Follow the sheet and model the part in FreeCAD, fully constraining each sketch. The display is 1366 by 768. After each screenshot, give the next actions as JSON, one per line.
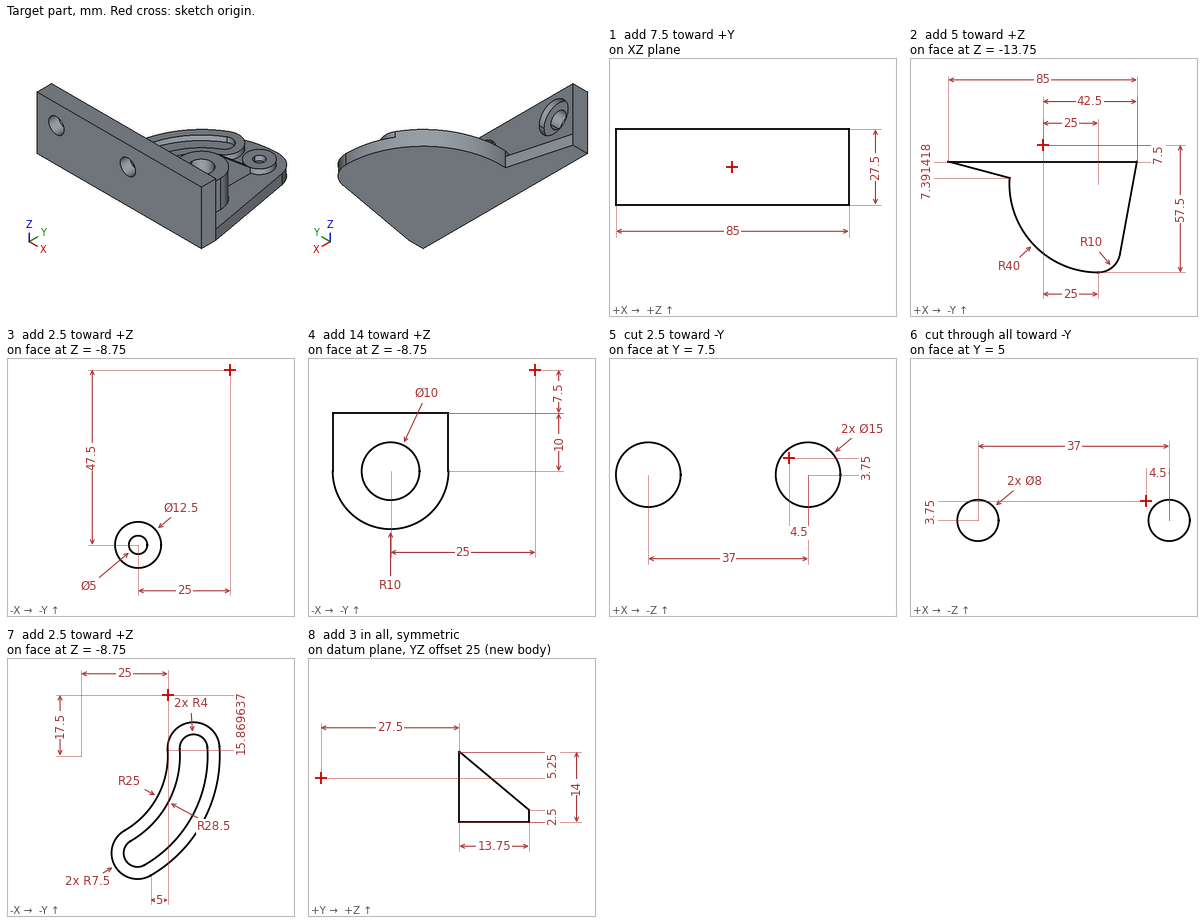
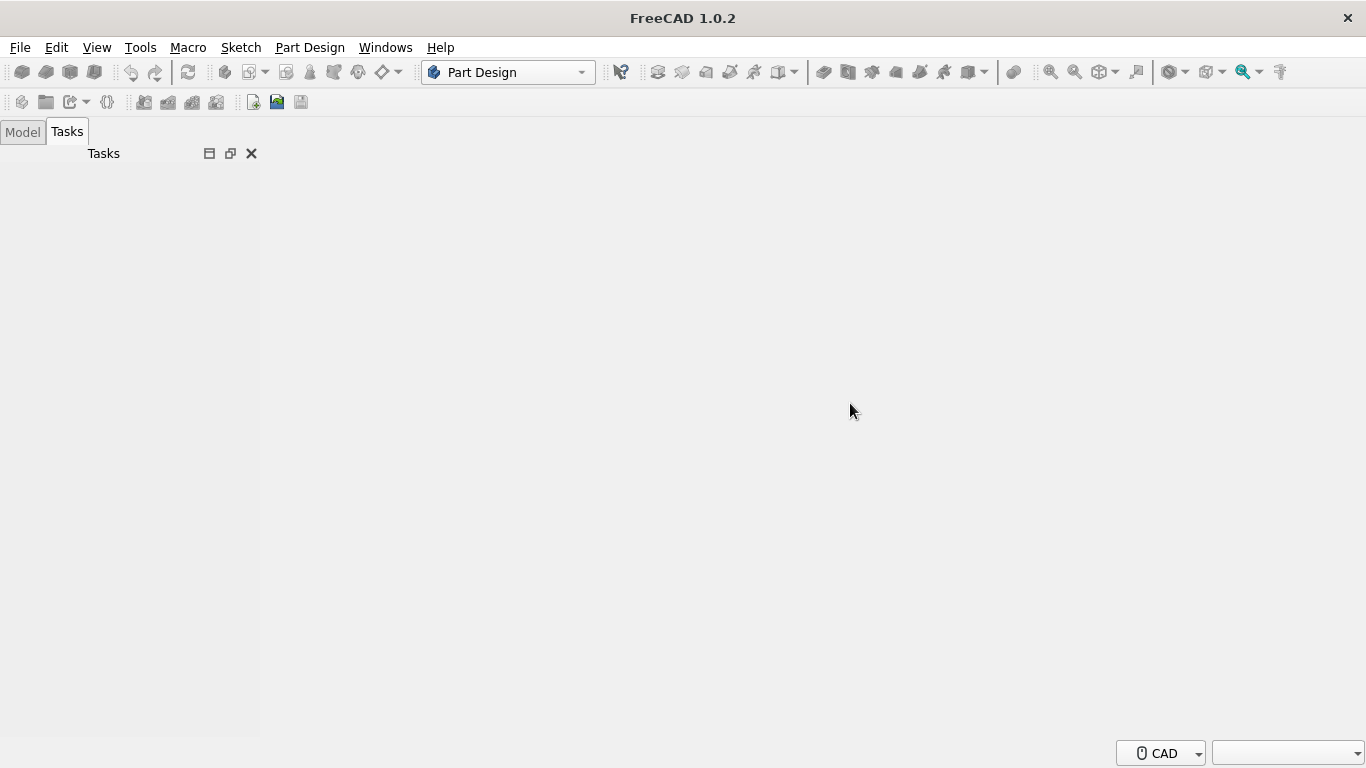
{"action": "left_click", "coordinate": [254, 102]}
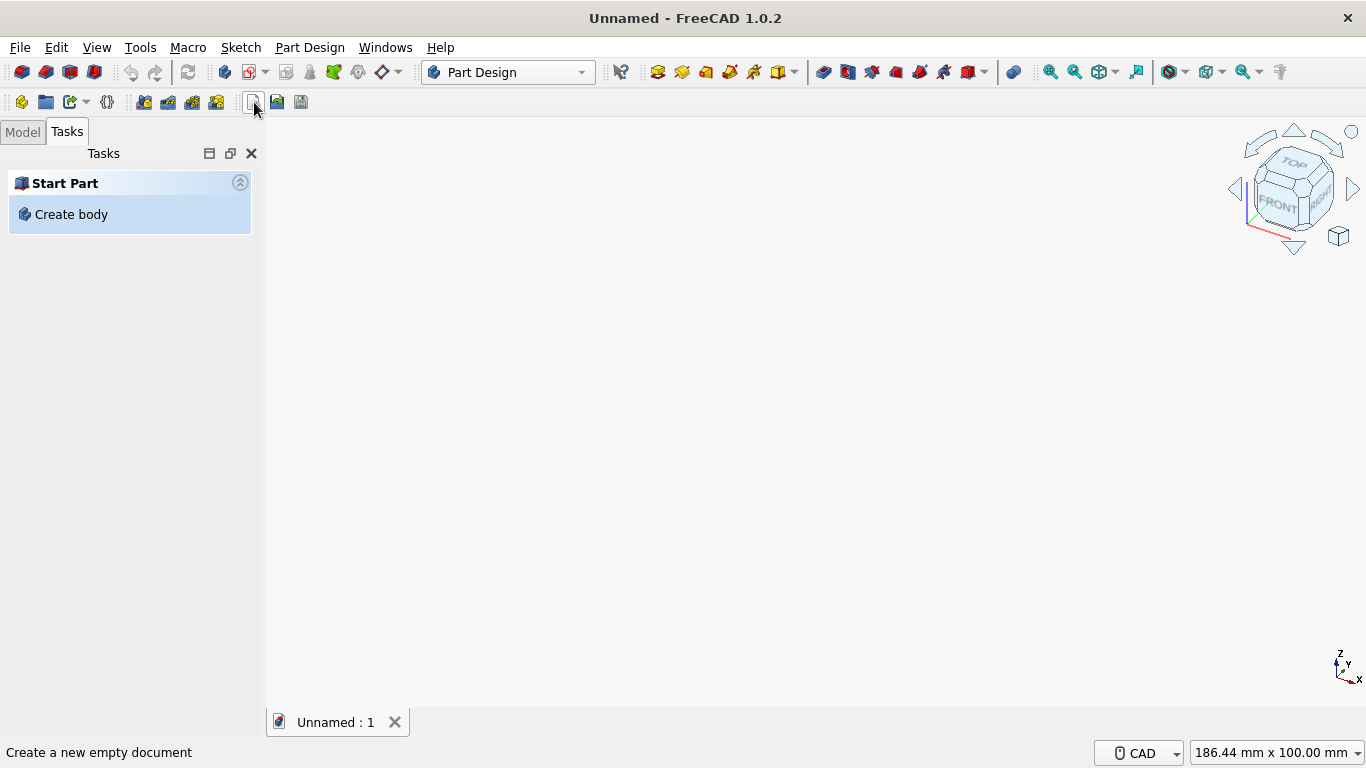
{"action": "left_click", "coordinate": [250, 72]}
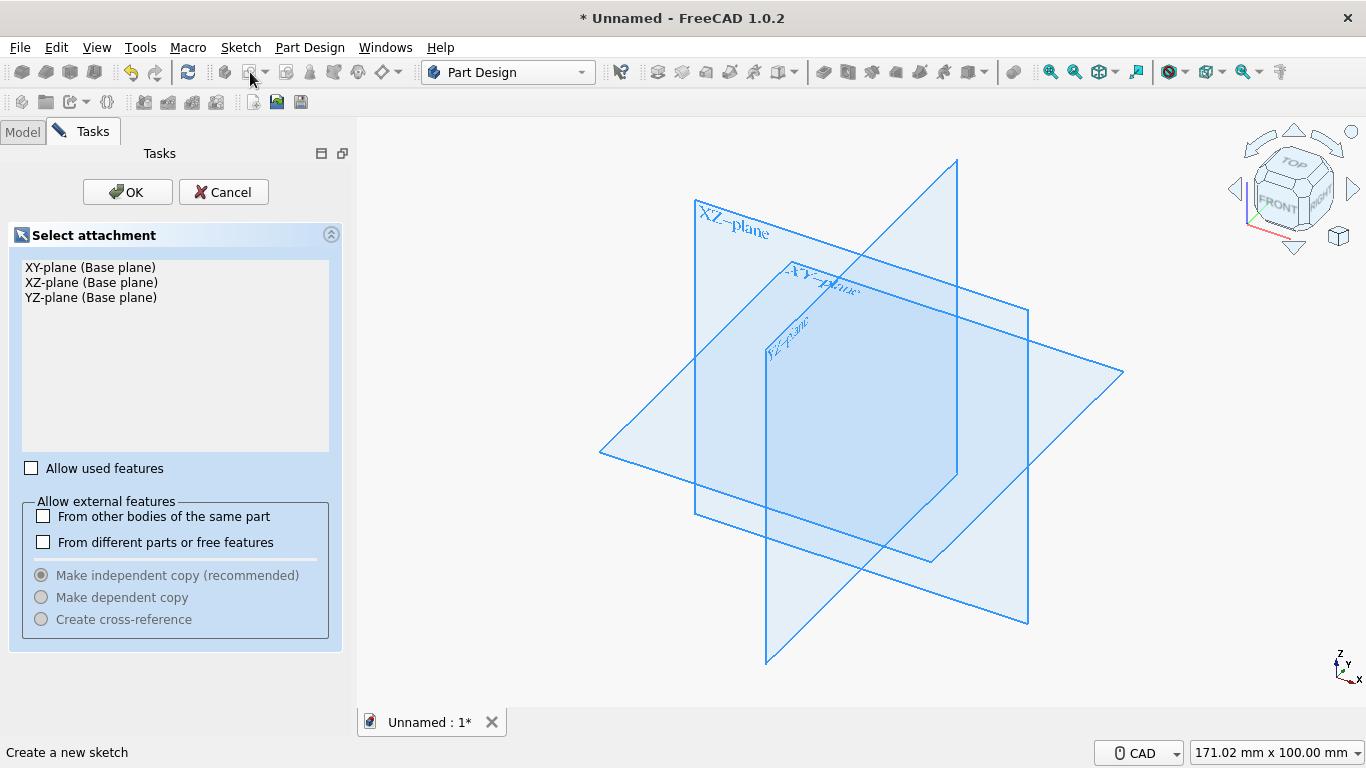
{"action": "left_click", "coordinate": [82, 282]}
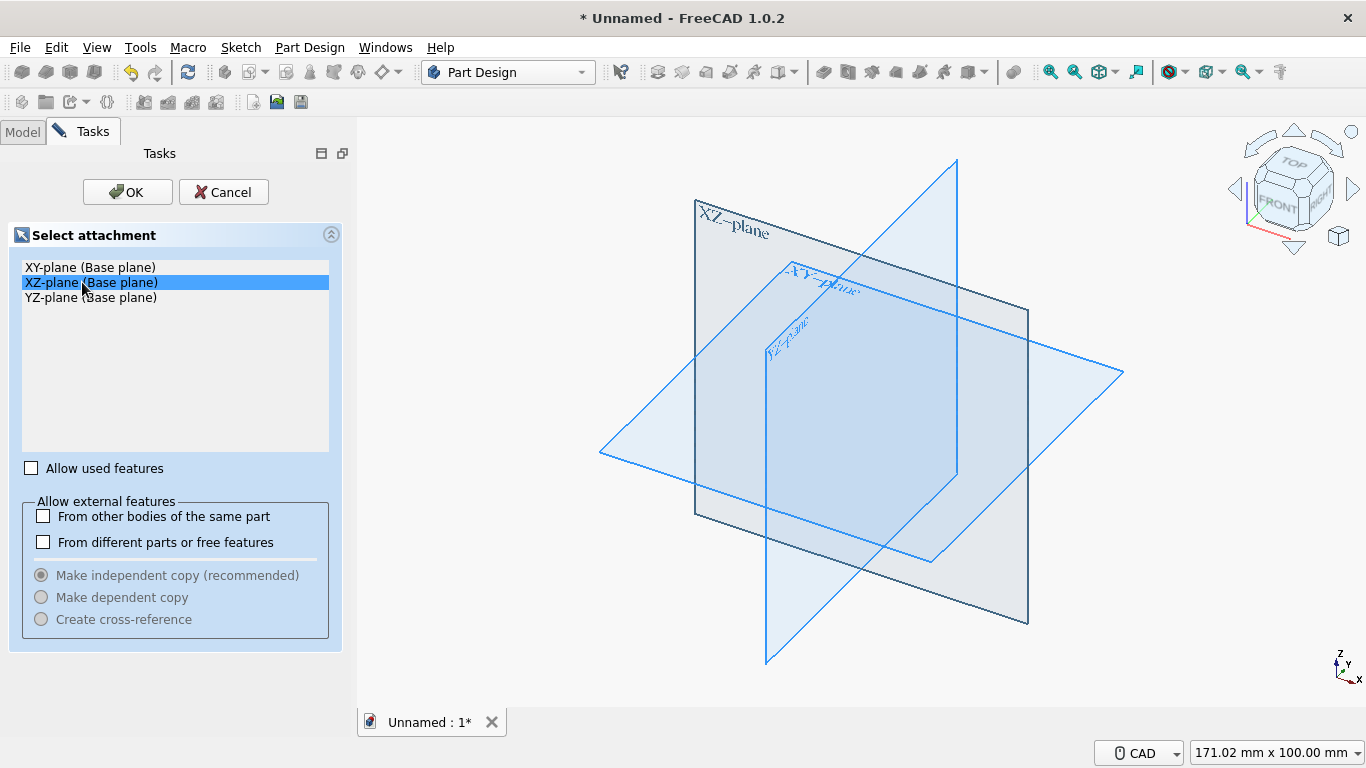
{"action": "left_click", "coordinate": [128, 192]}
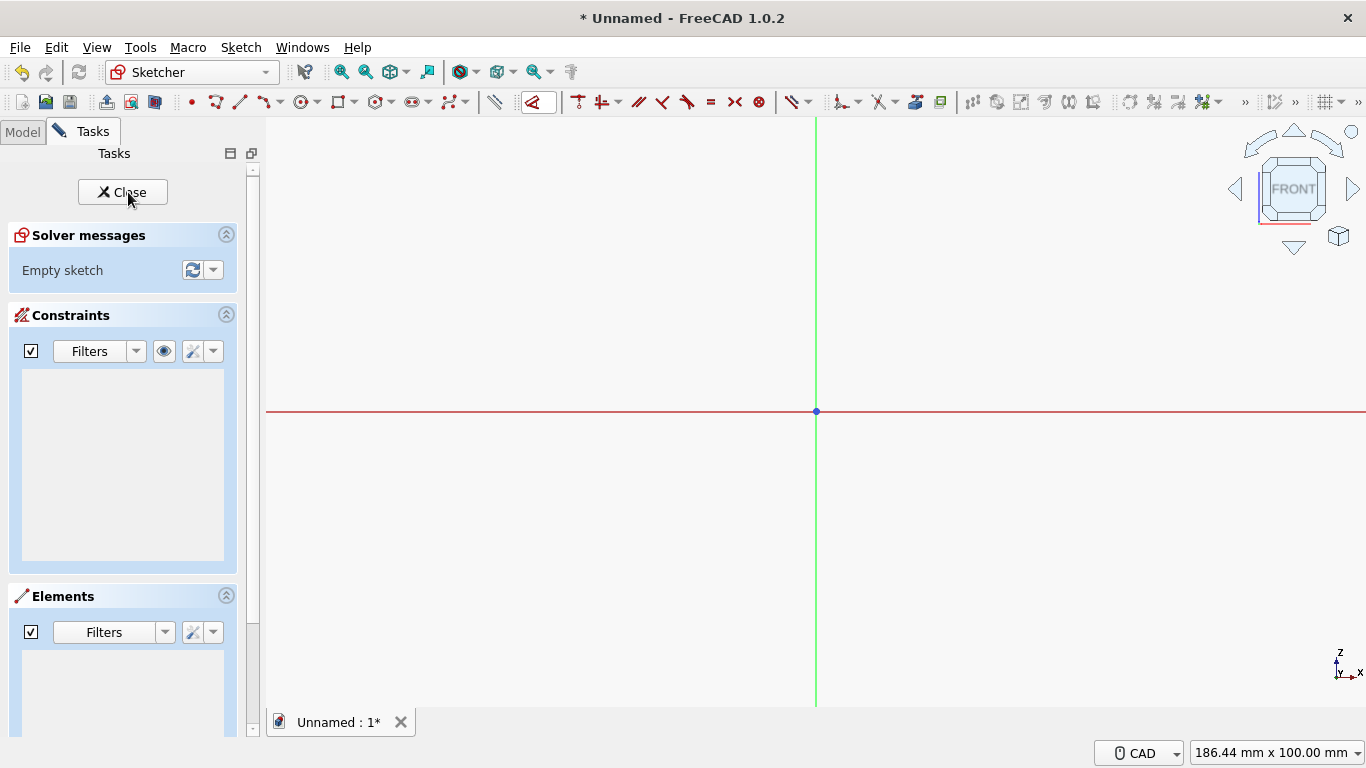
{"action": "left_click", "coordinate": [356, 102]}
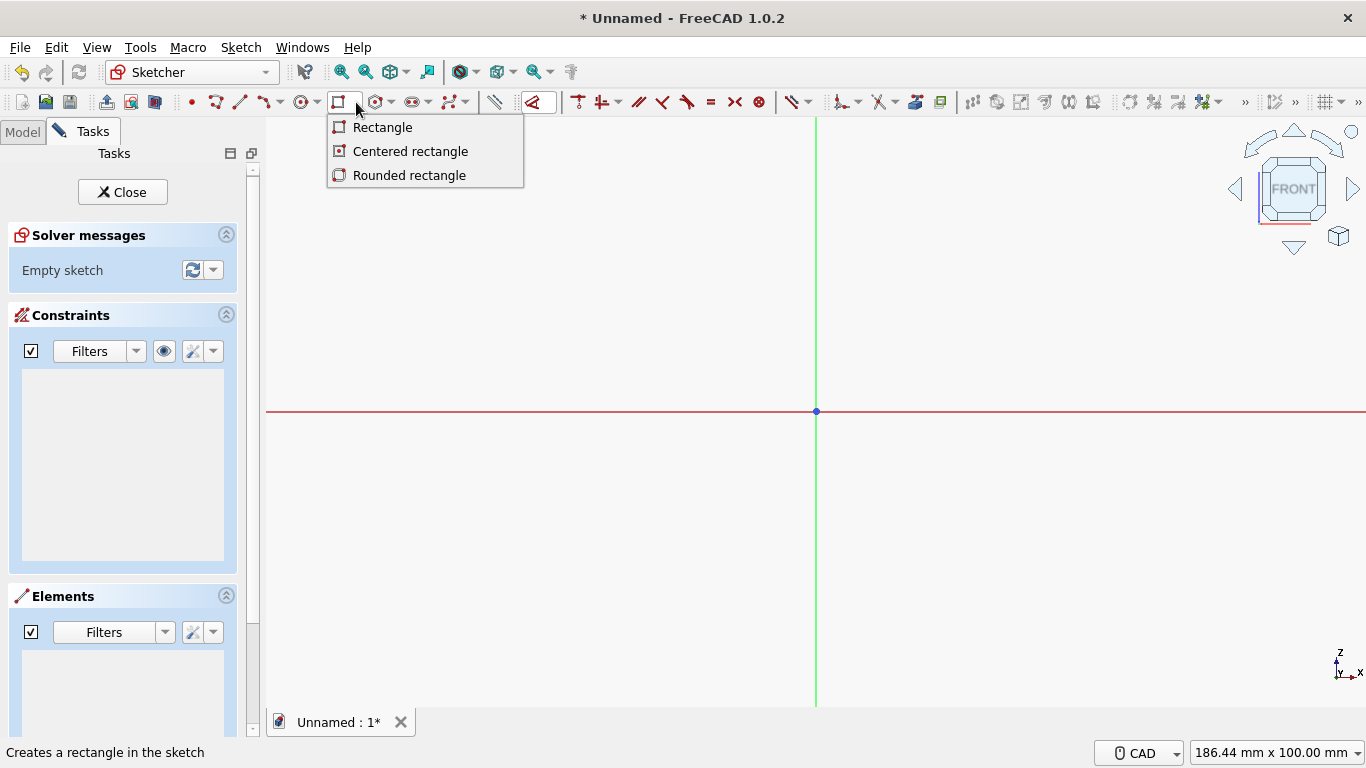
{"action": "left_click", "coordinate": [426, 151]}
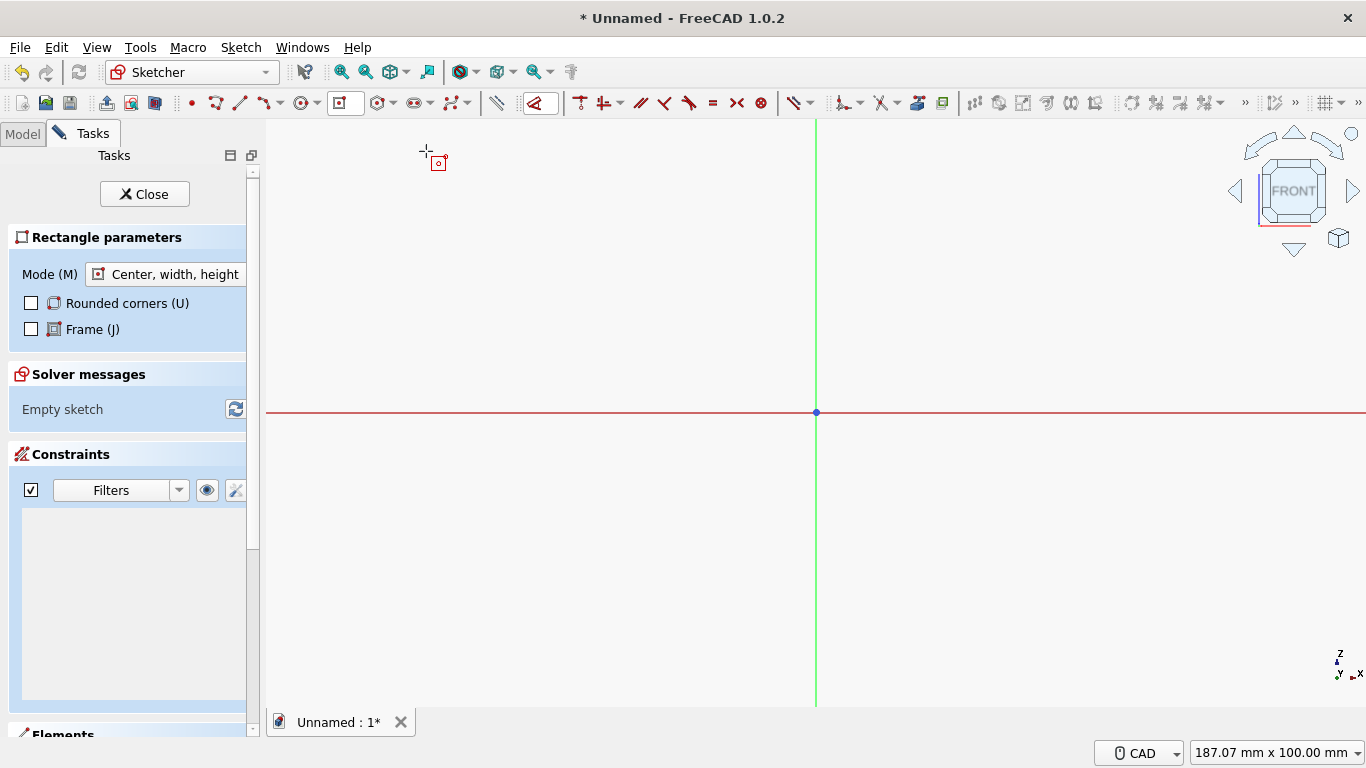
{"action": "left_click", "coordinate": [816, 413]}
{"action": "mouse_move", "coordinate": [1066, 332]}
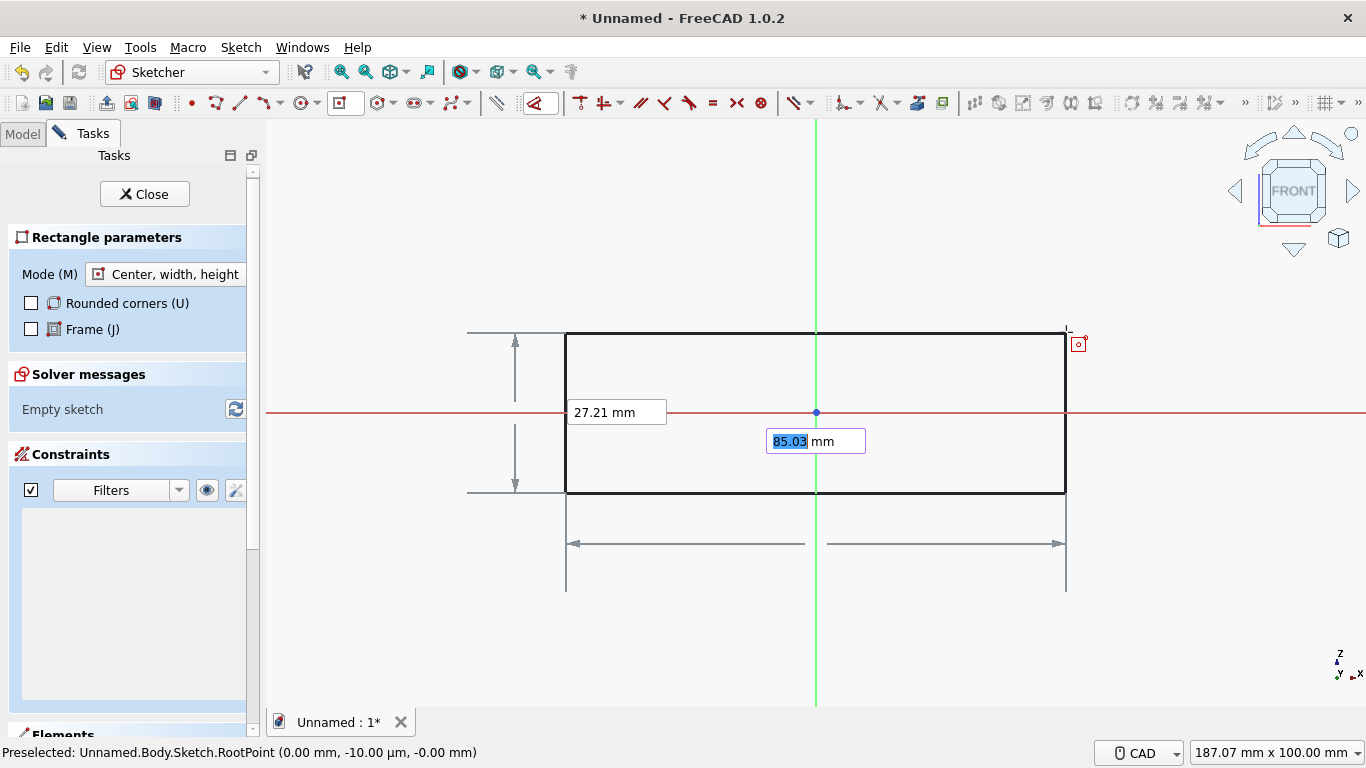
{"action": "type", "text": "85"}
{"action": "key", "text": "Tab"}
{"action": "type", "text": "27.5"}
{"action": "key", "text": "Return"}
{"action": "key", "text": "Escape"}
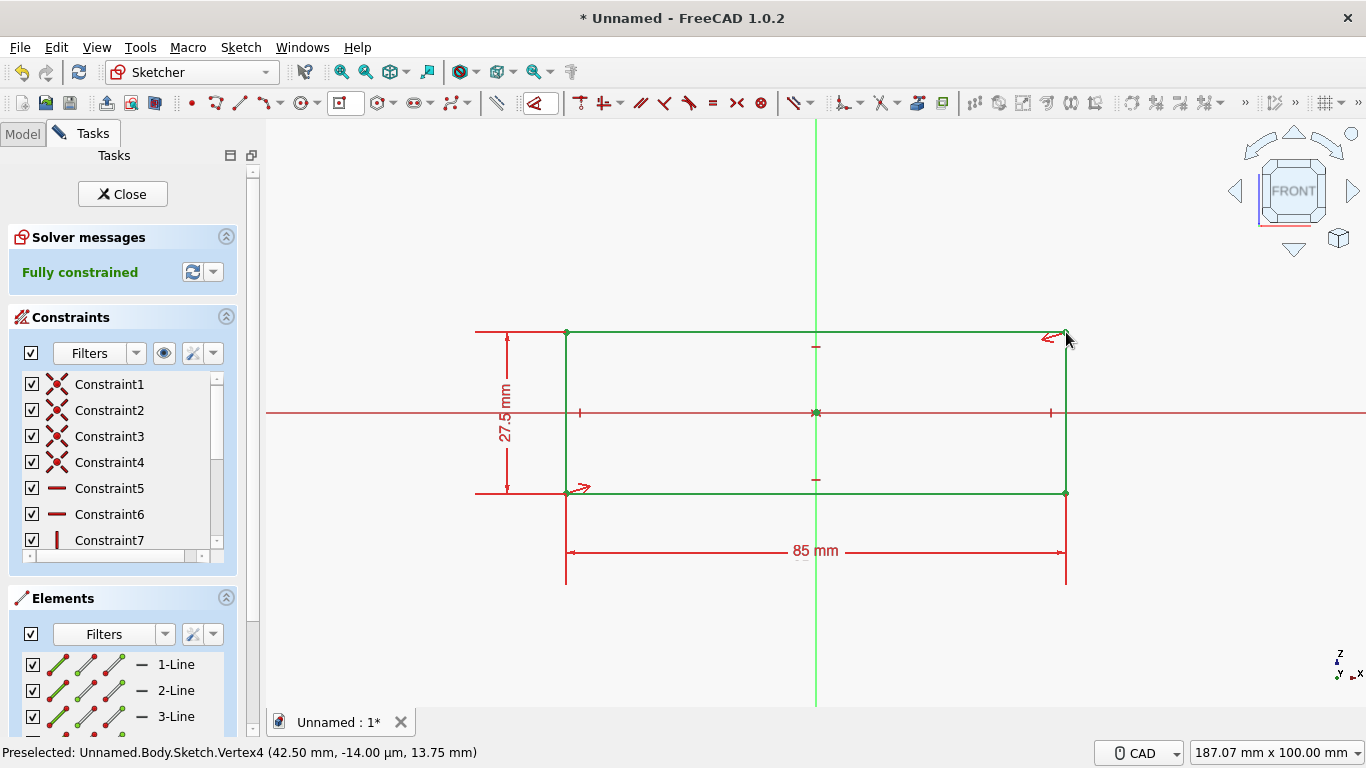
{"action": "left_click", "coordinate": [123, 194]}